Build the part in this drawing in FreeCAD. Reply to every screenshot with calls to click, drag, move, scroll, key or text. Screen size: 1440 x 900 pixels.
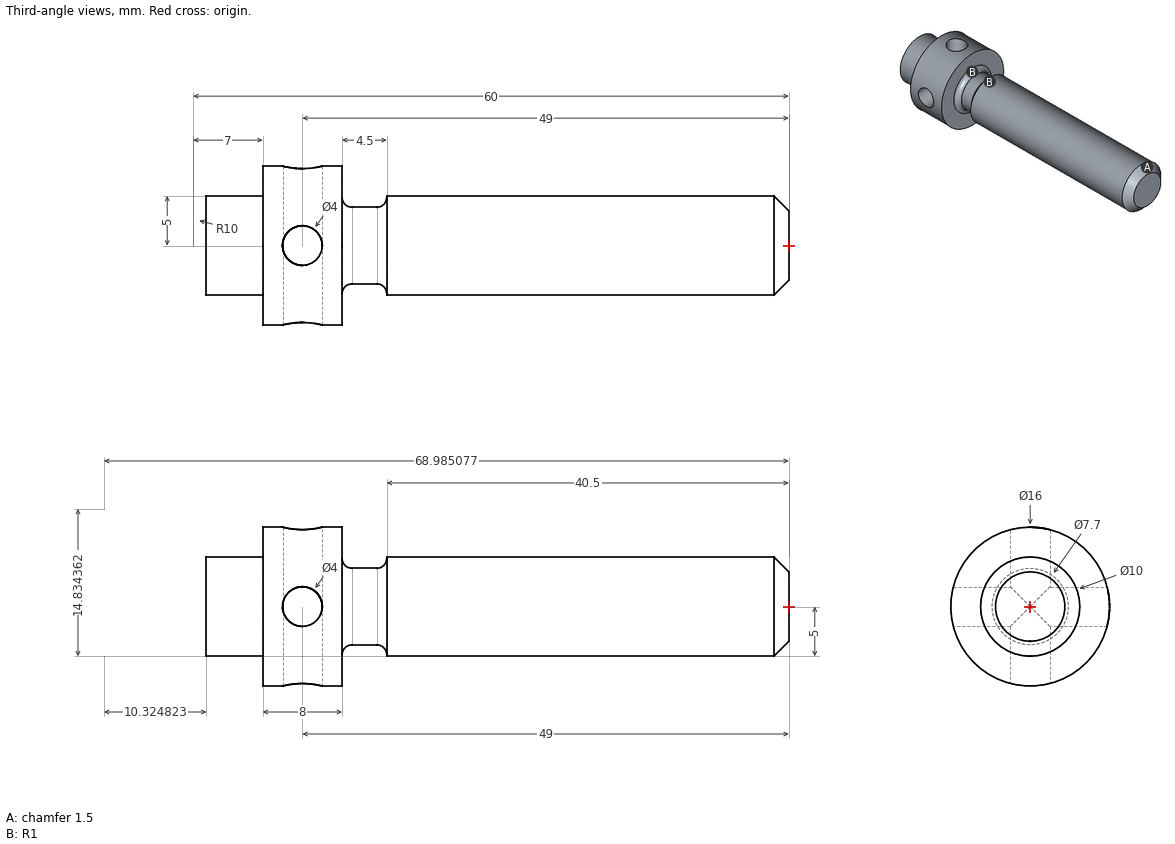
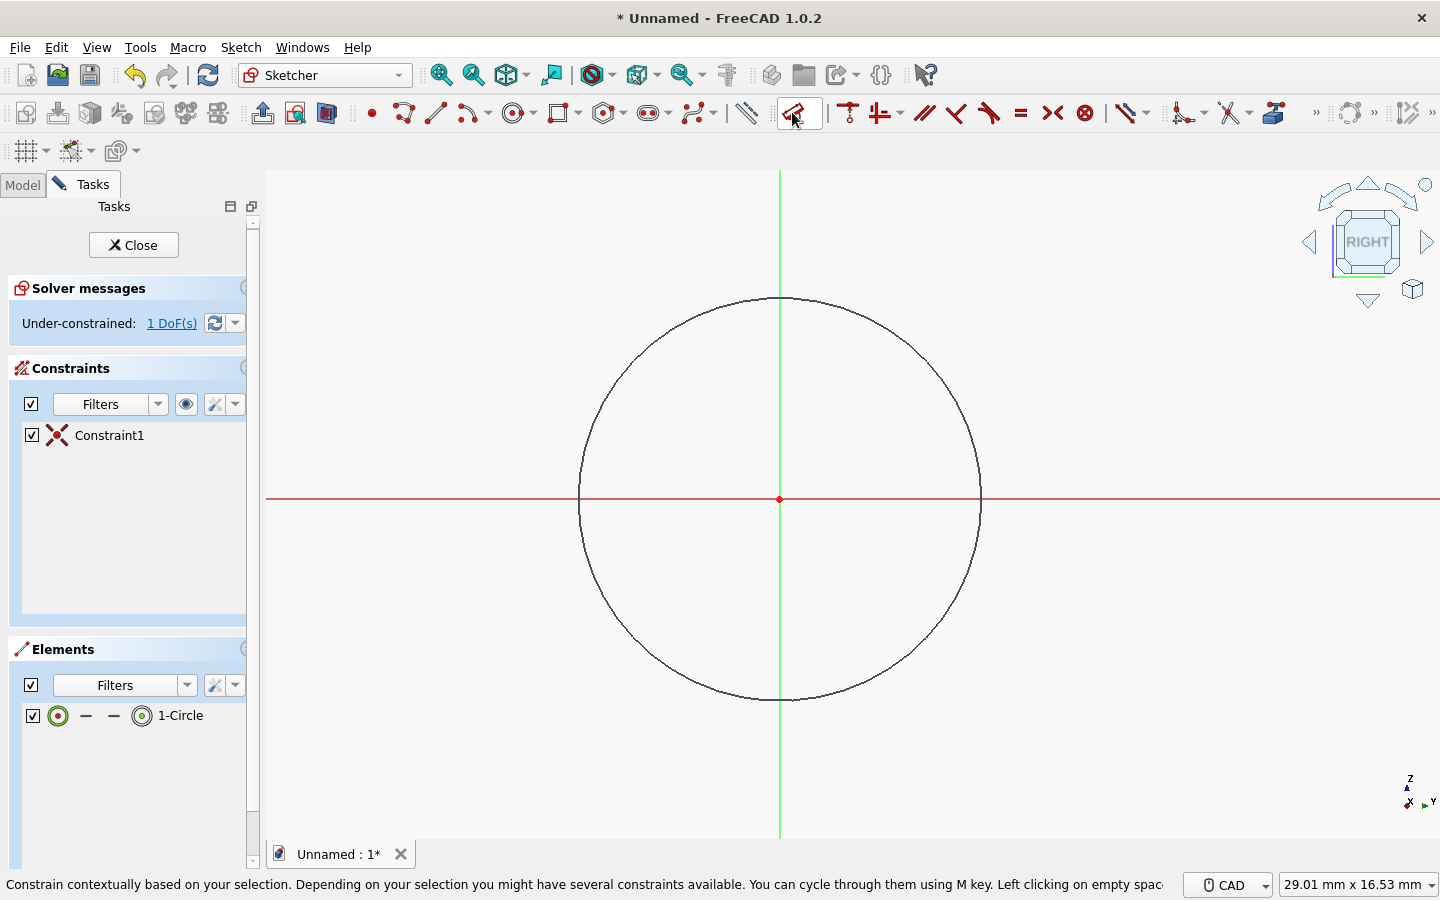
click(922, 357)
click(945, 334)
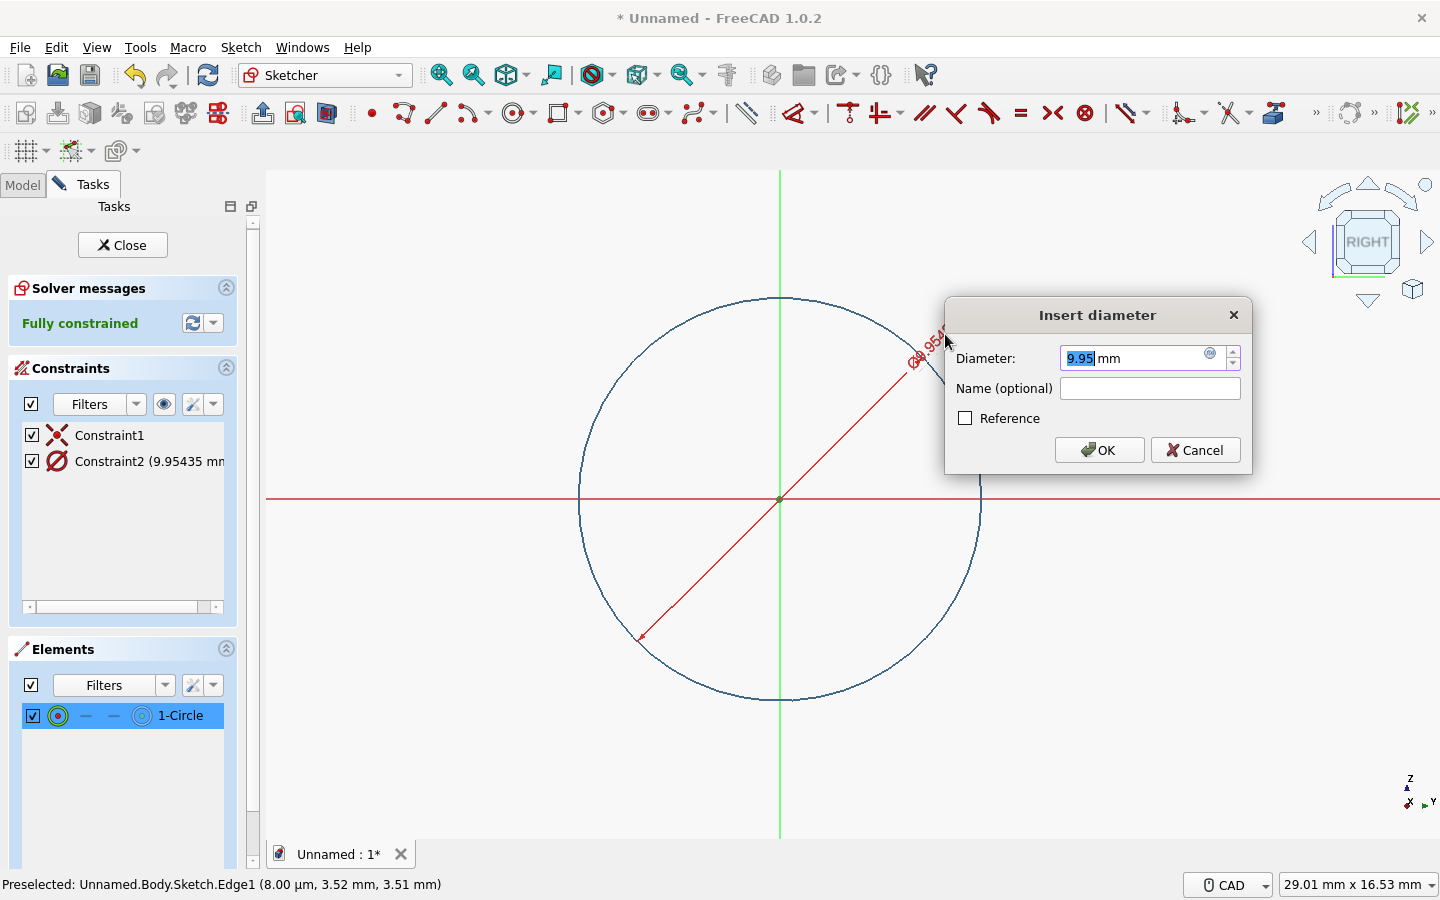
text(10)
key(Return)
key(Escape)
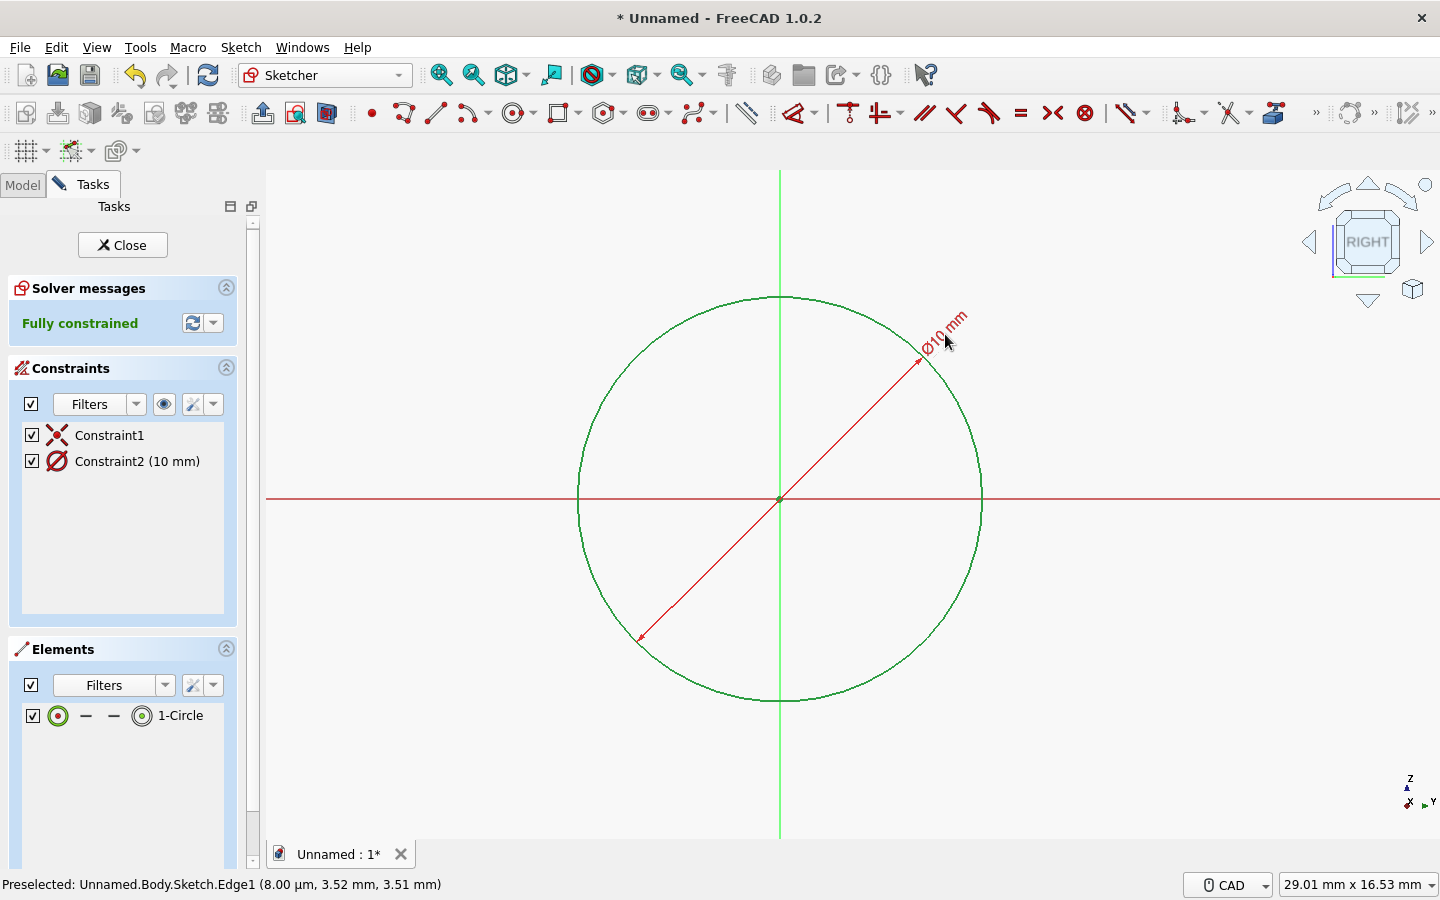
click(123, 245)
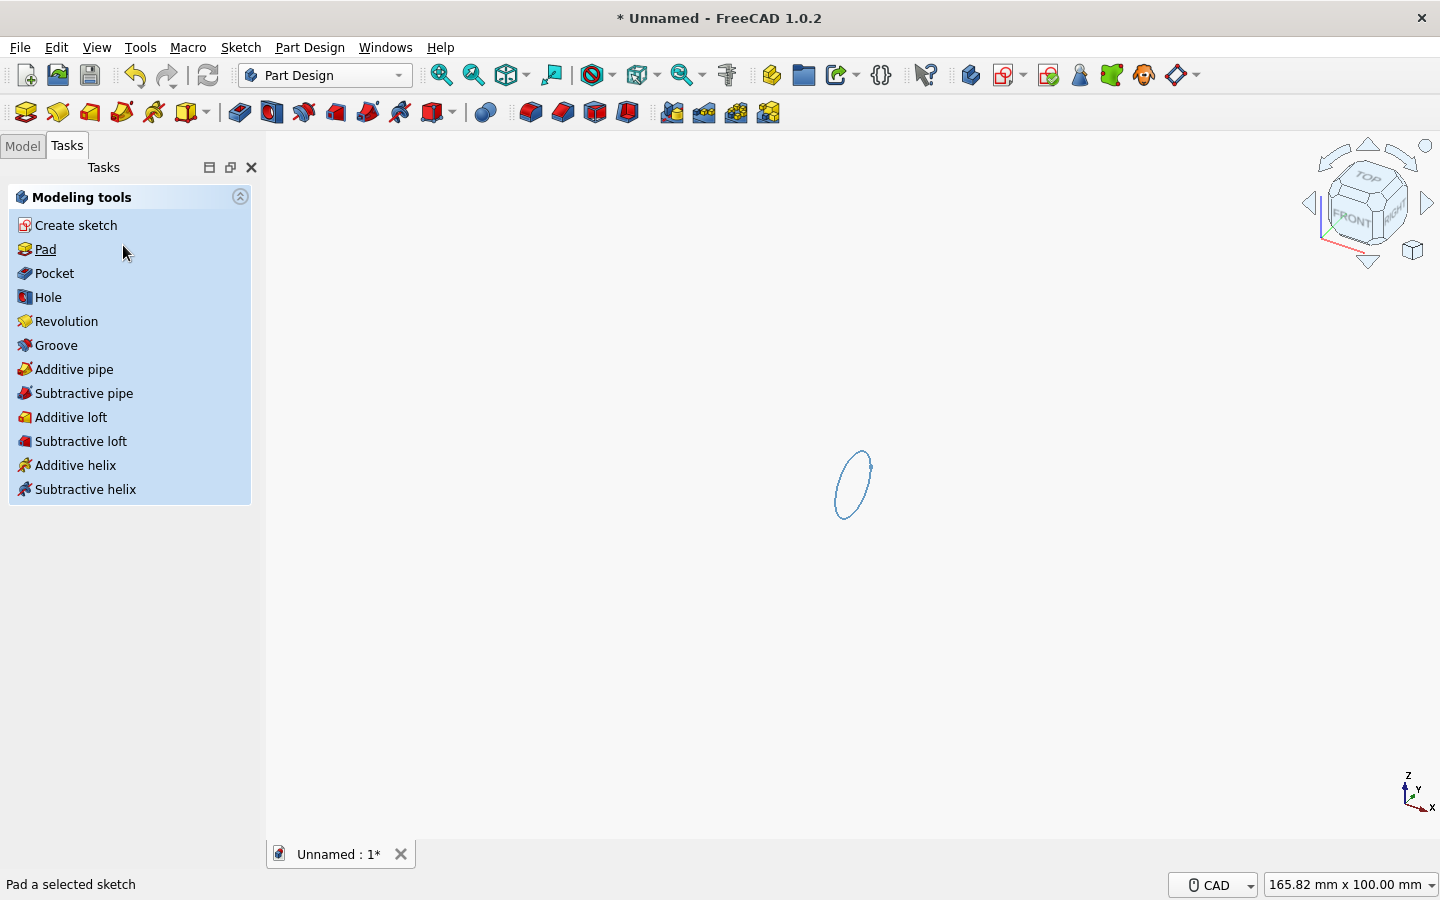
click(26, 112)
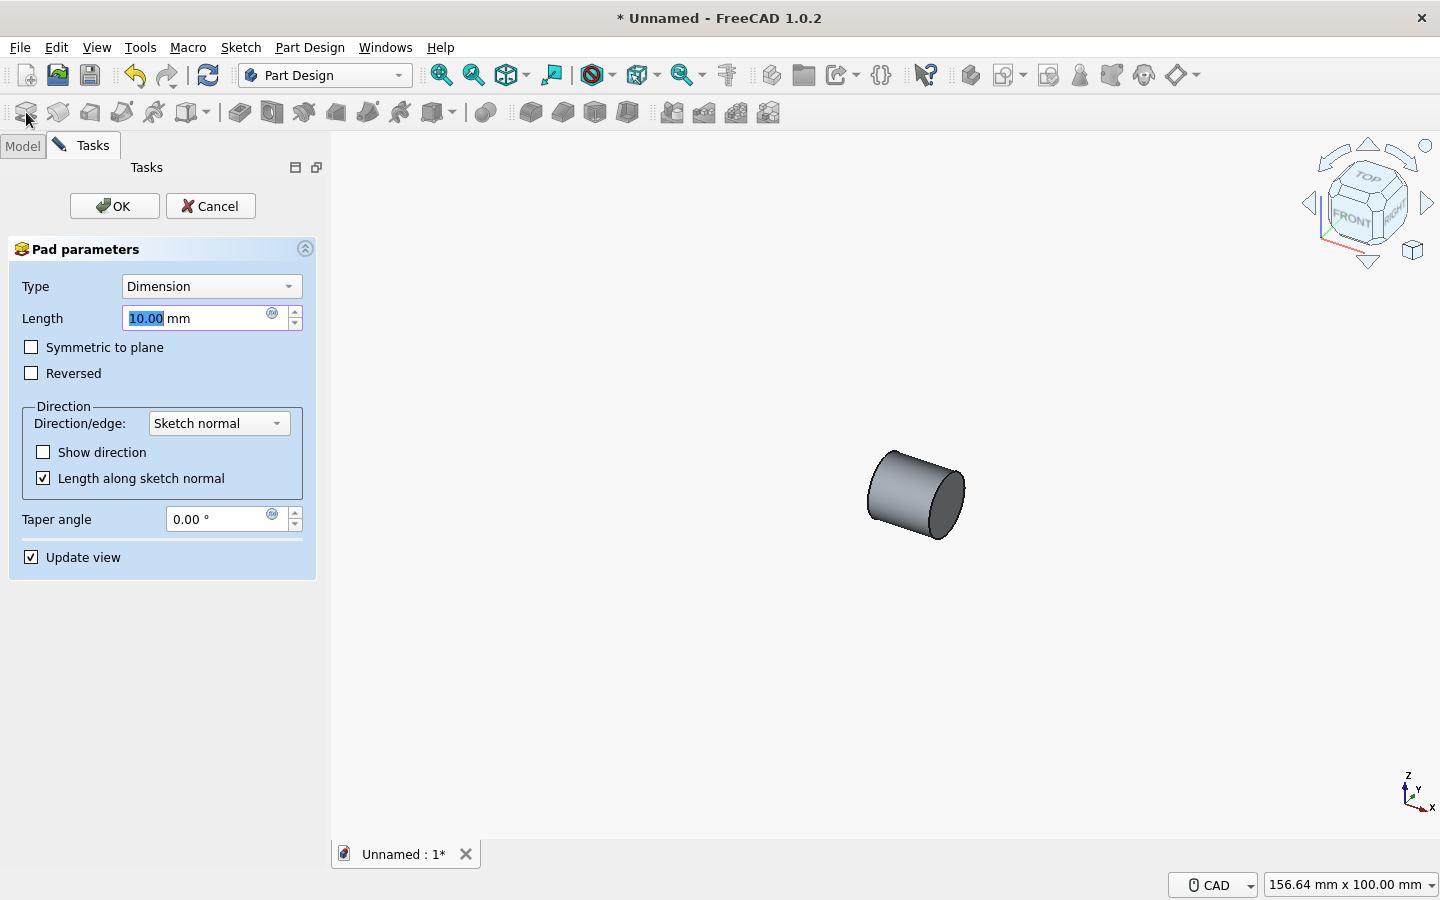
text(40.5)
key(Tab)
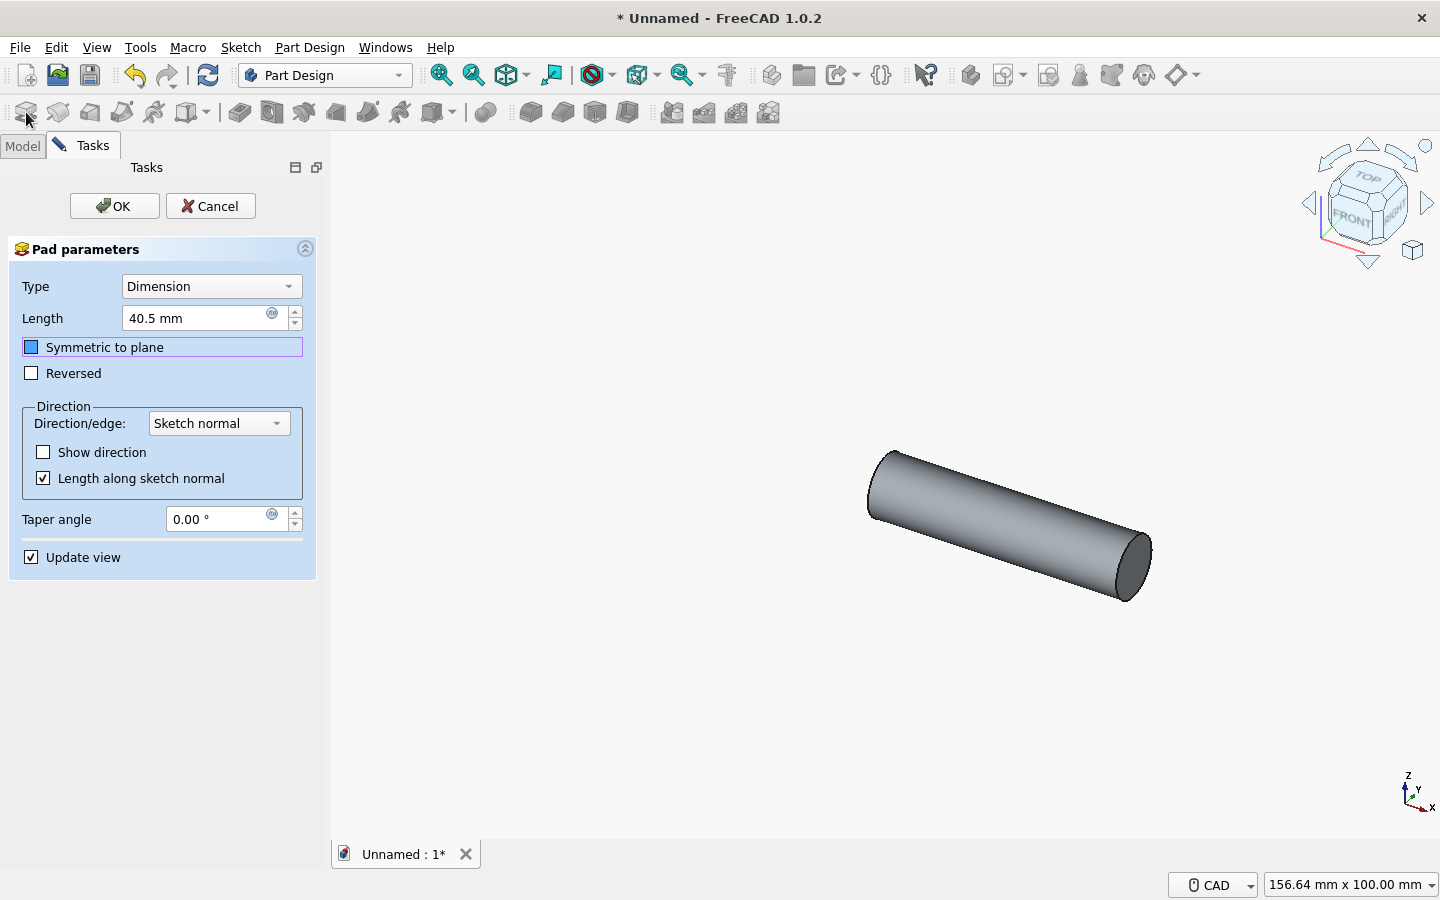
click(30, 373)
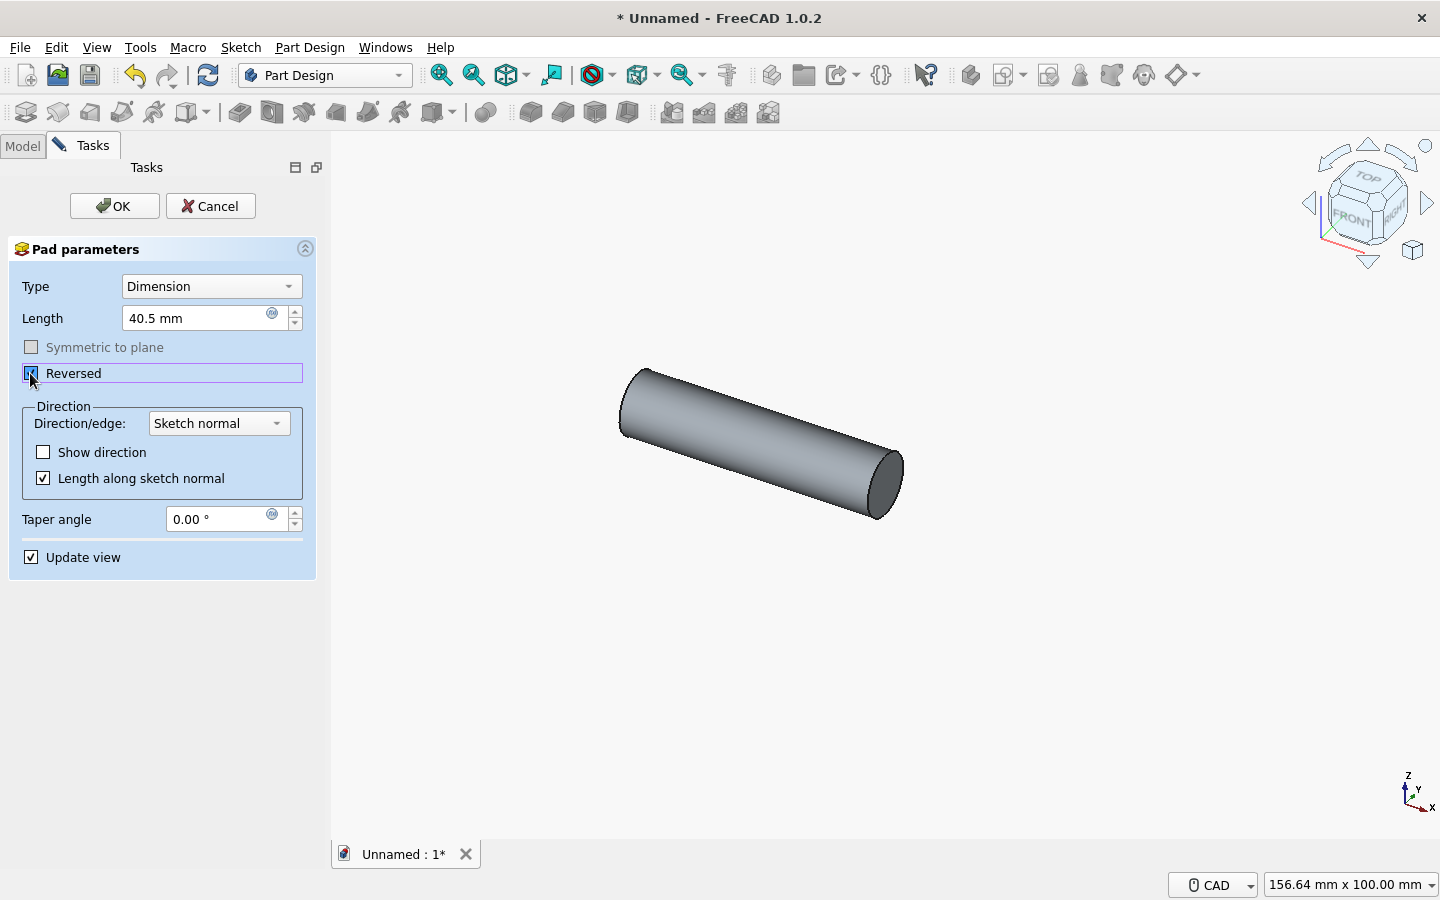
click(115, 206)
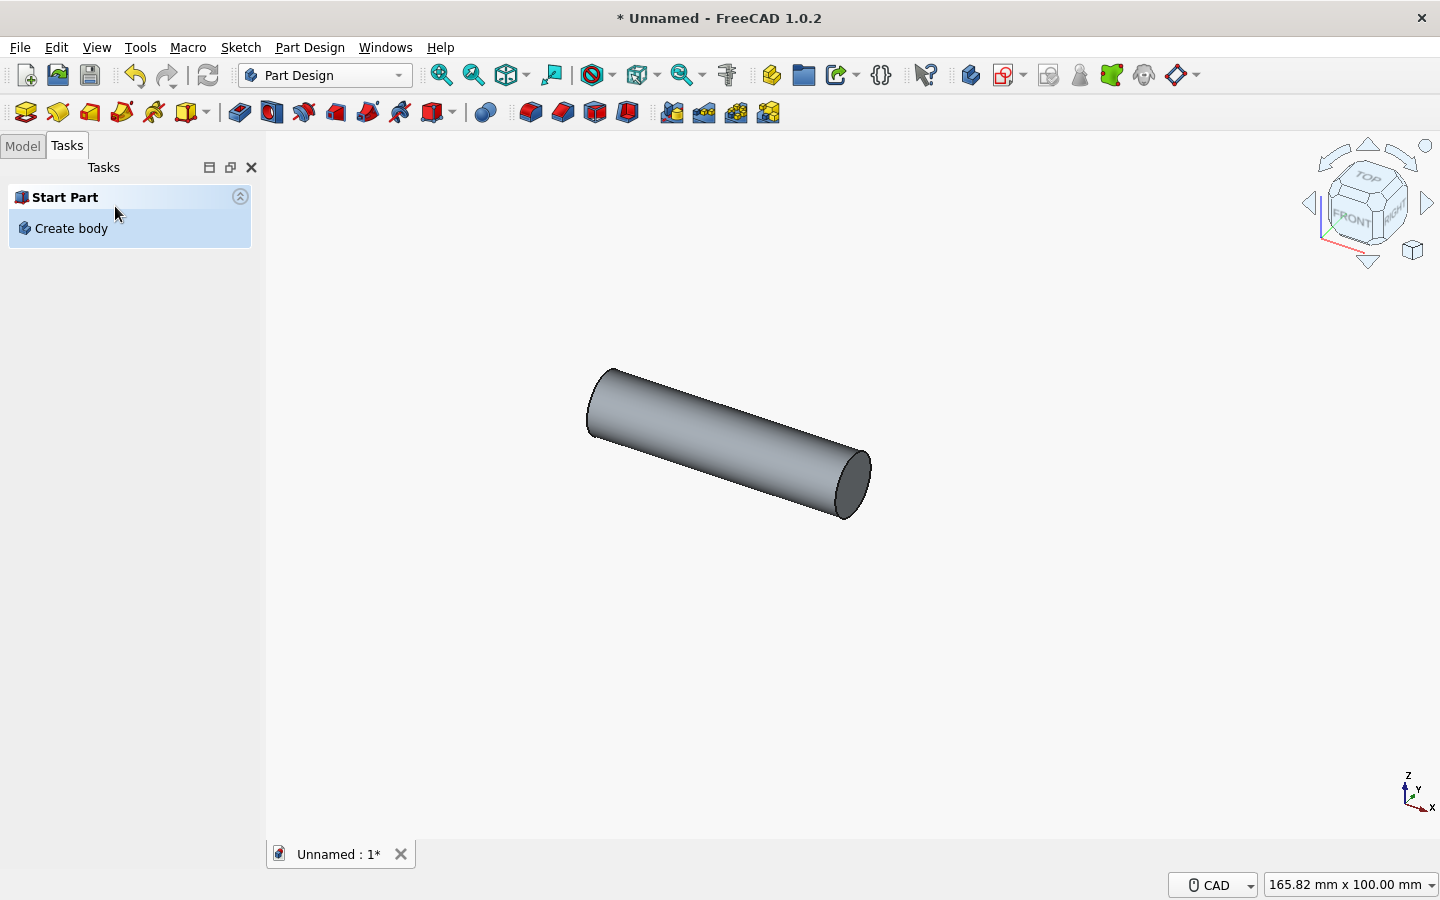
key(v)
key(f)